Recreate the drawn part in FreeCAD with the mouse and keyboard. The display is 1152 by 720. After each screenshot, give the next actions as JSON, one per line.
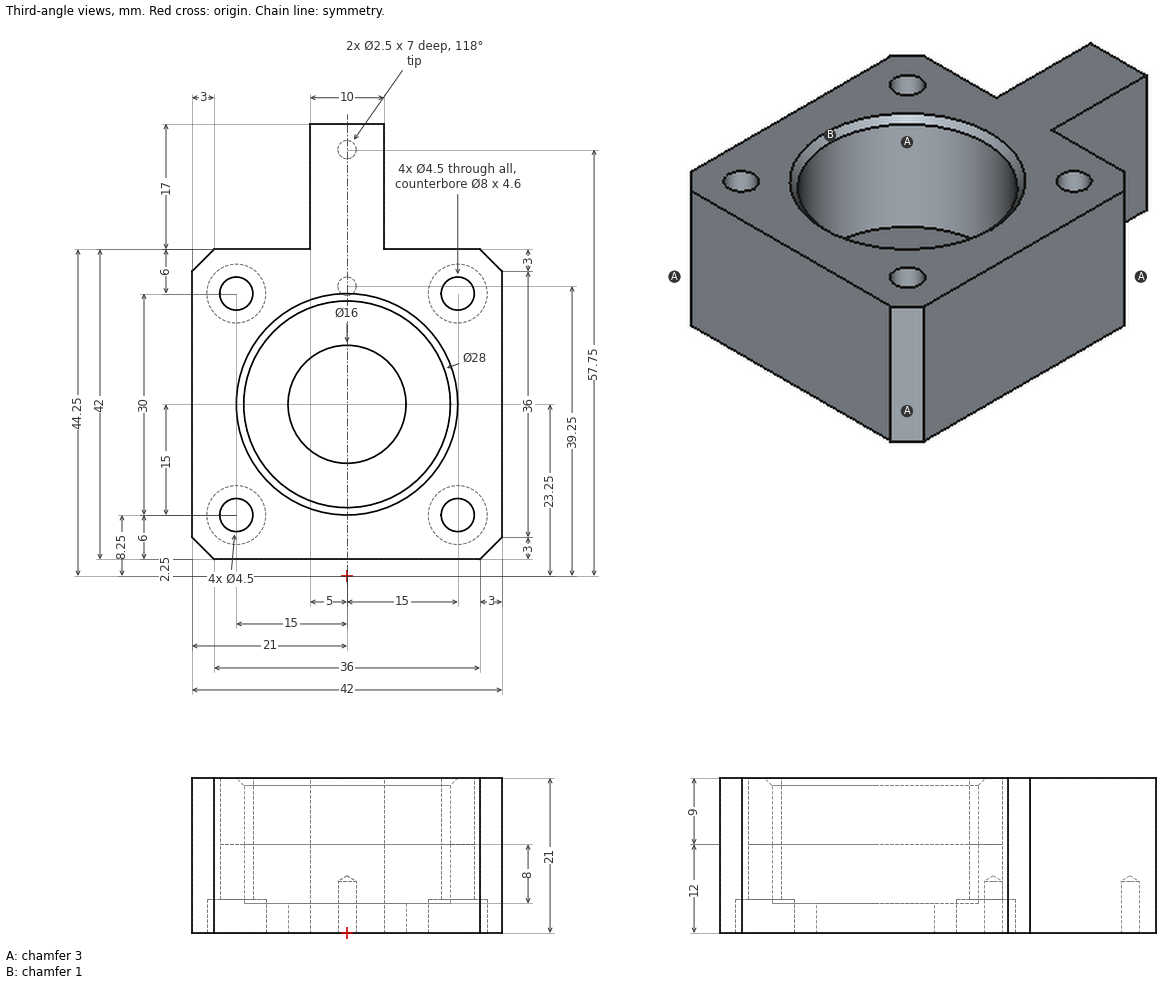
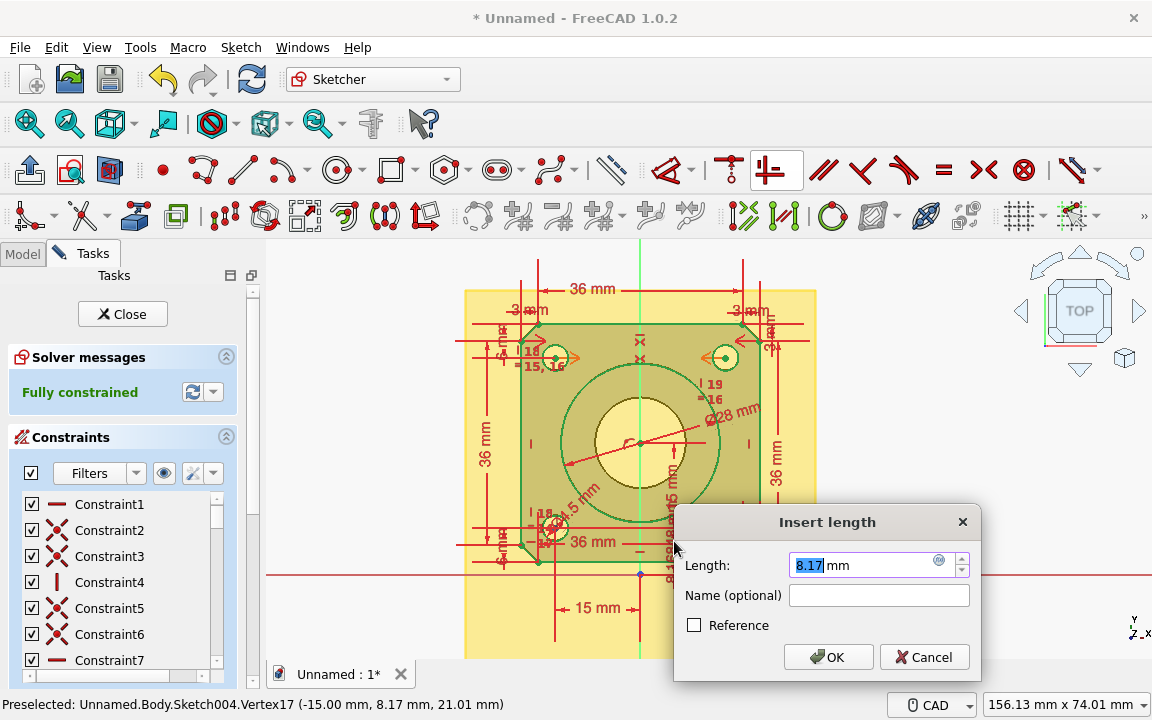
{"action": "type", "text": "8.25"}
{"action": "key", "text": "Return"}
{"action": "key", "text": "Escape"}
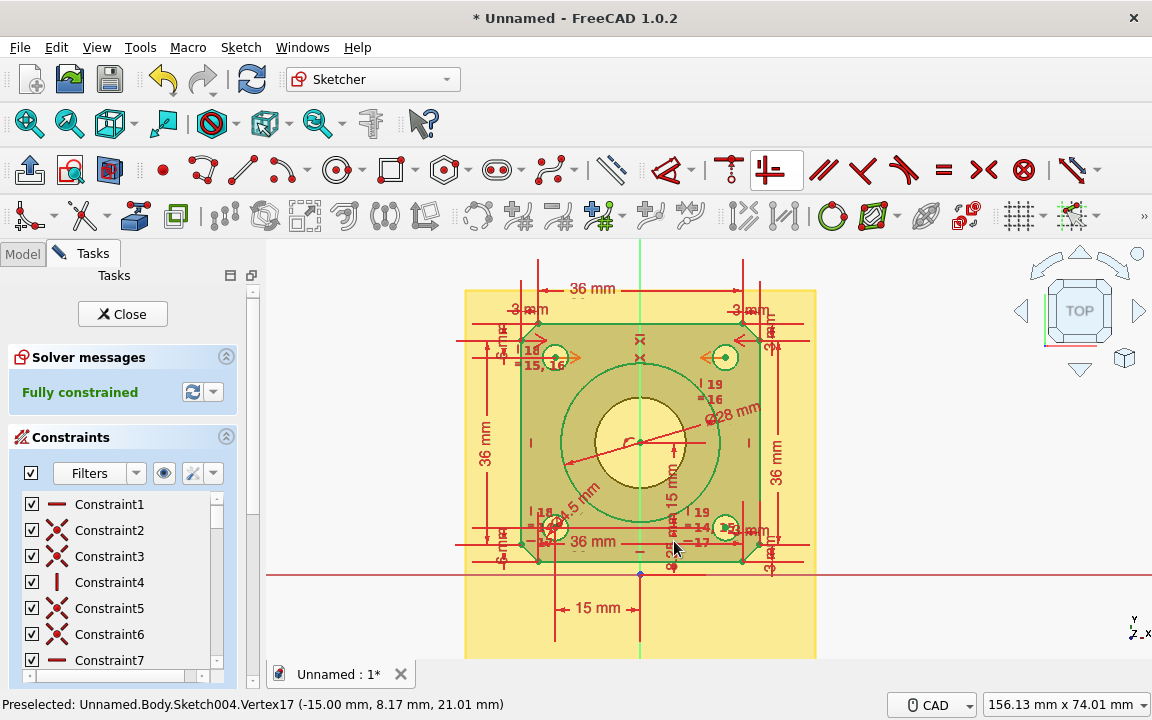
{"action": "left_click", "coordinate": [123, 314]}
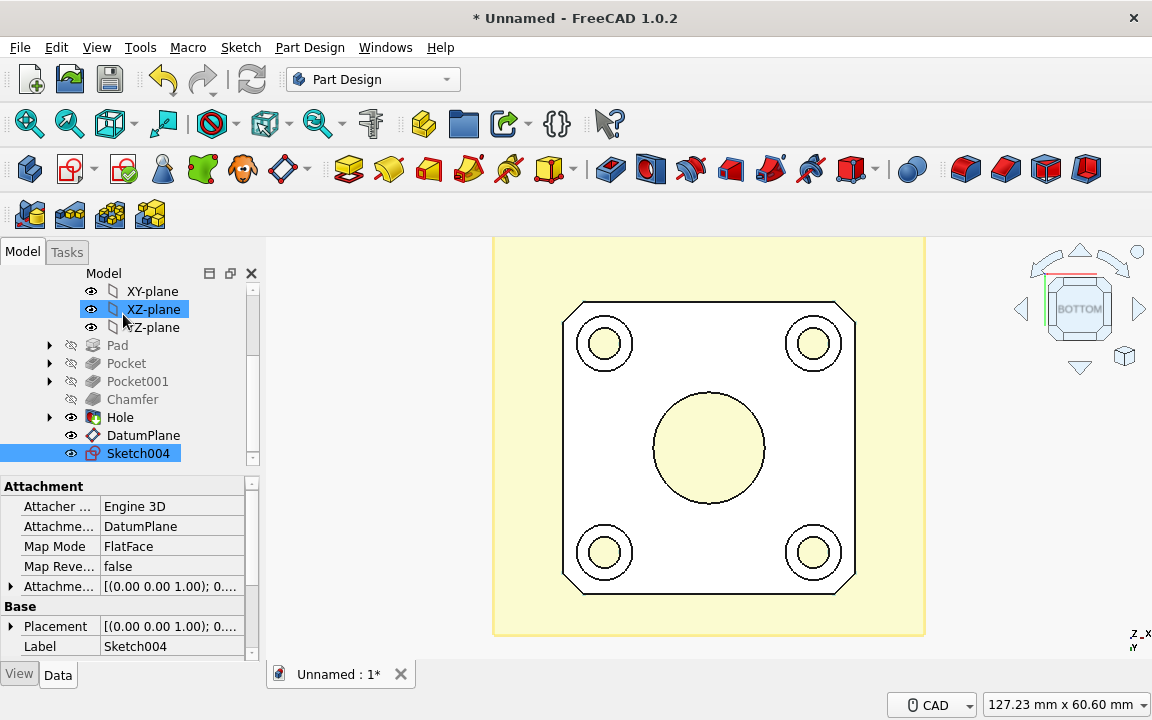
{"action": "left_click", "coordinate": [350, 170]}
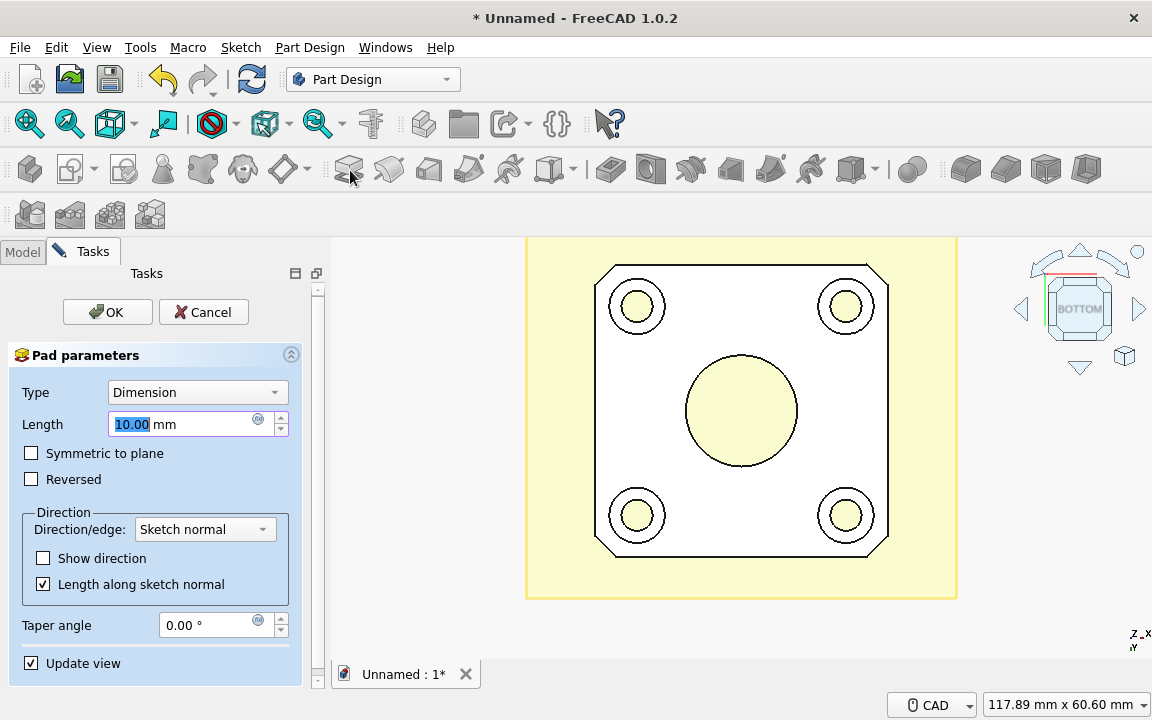
{"action": "type", "text": "9"}
{"action": "key", "text": "Tab"}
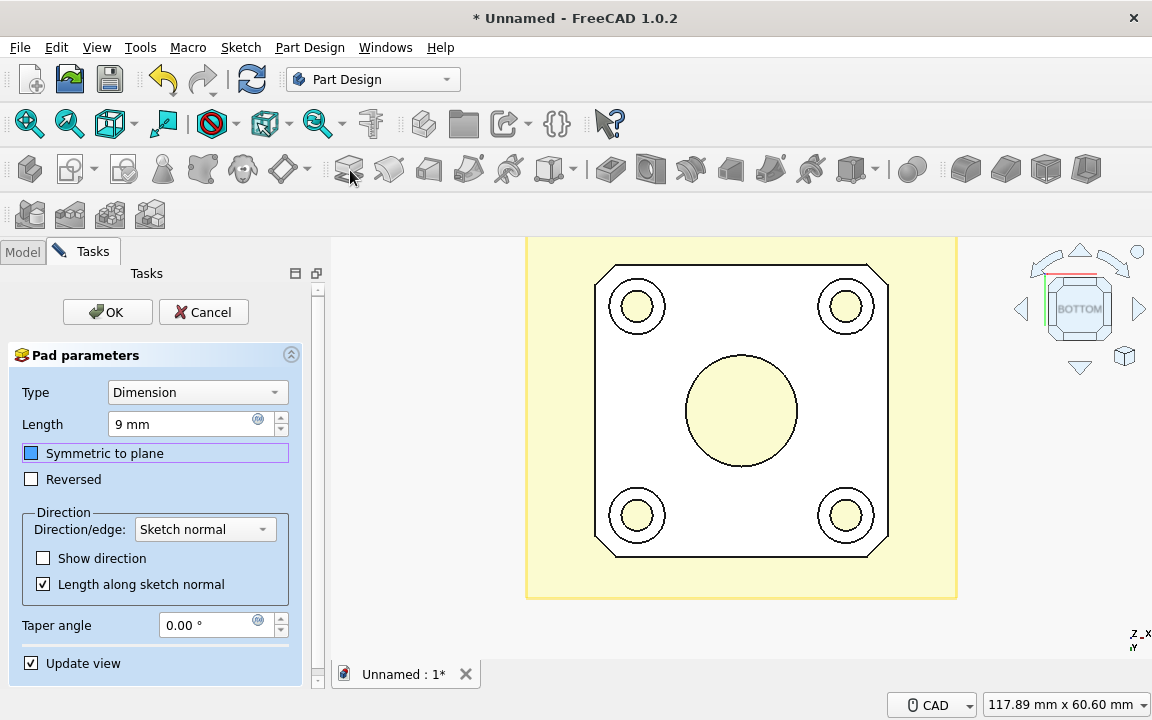
{"action": "left_click", "coordinate": [30, 479]}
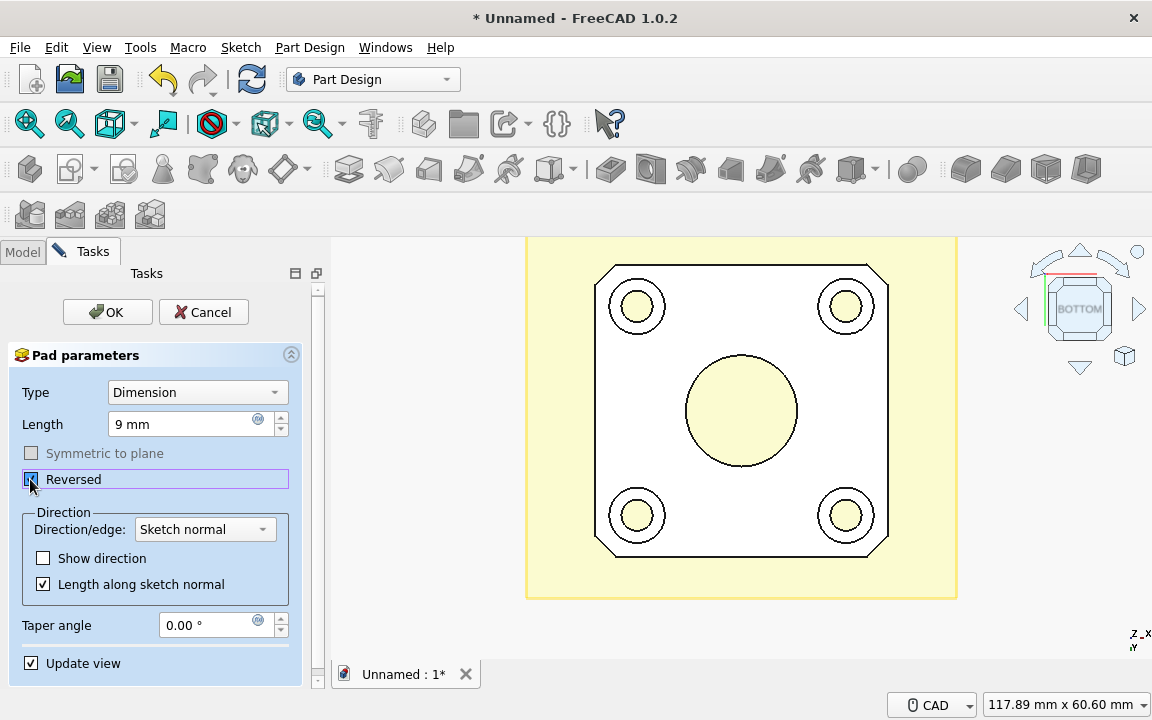
{"action": "left_click", "coordinate": [108, 312]}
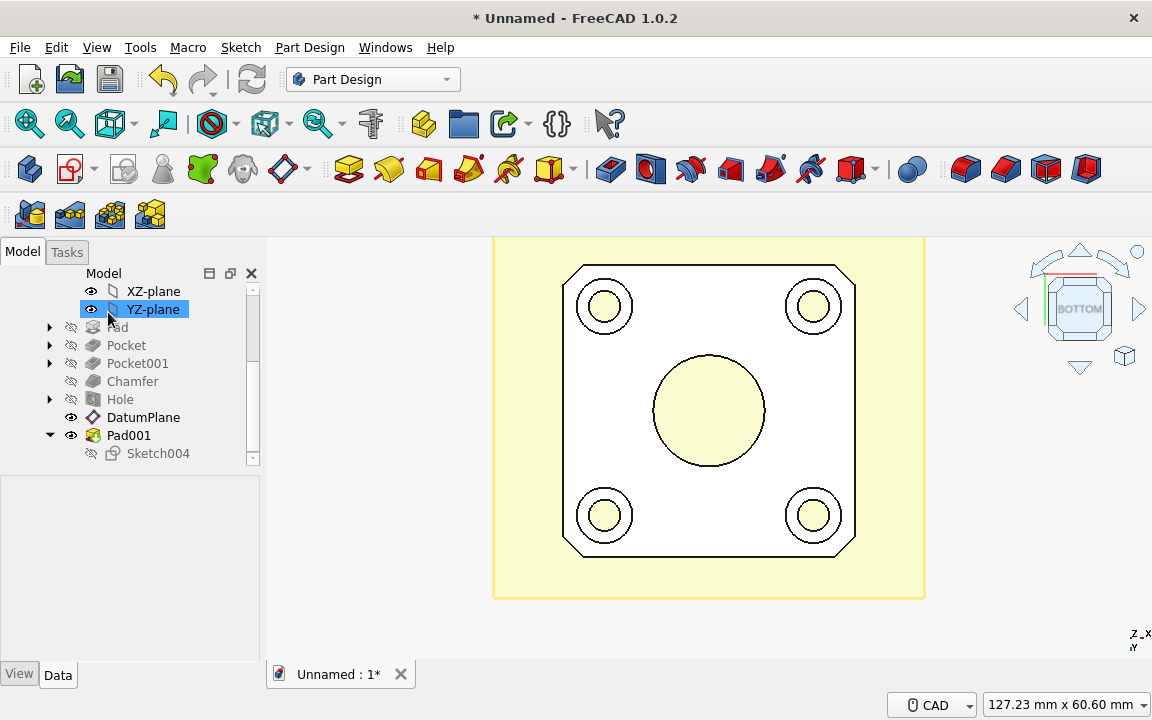
{"action": "left_click", "coordinate": [116, 417]}
{"action": "key", "text": "space"}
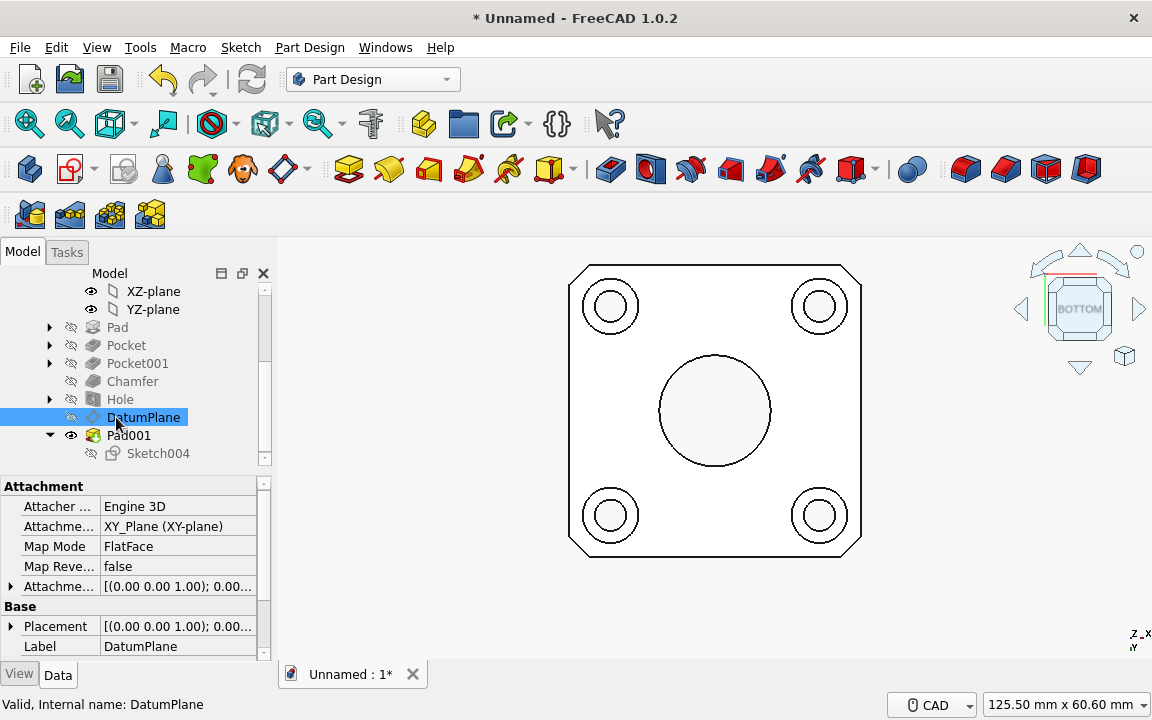
{"action": "left_click", "coordinate": [757, 326]}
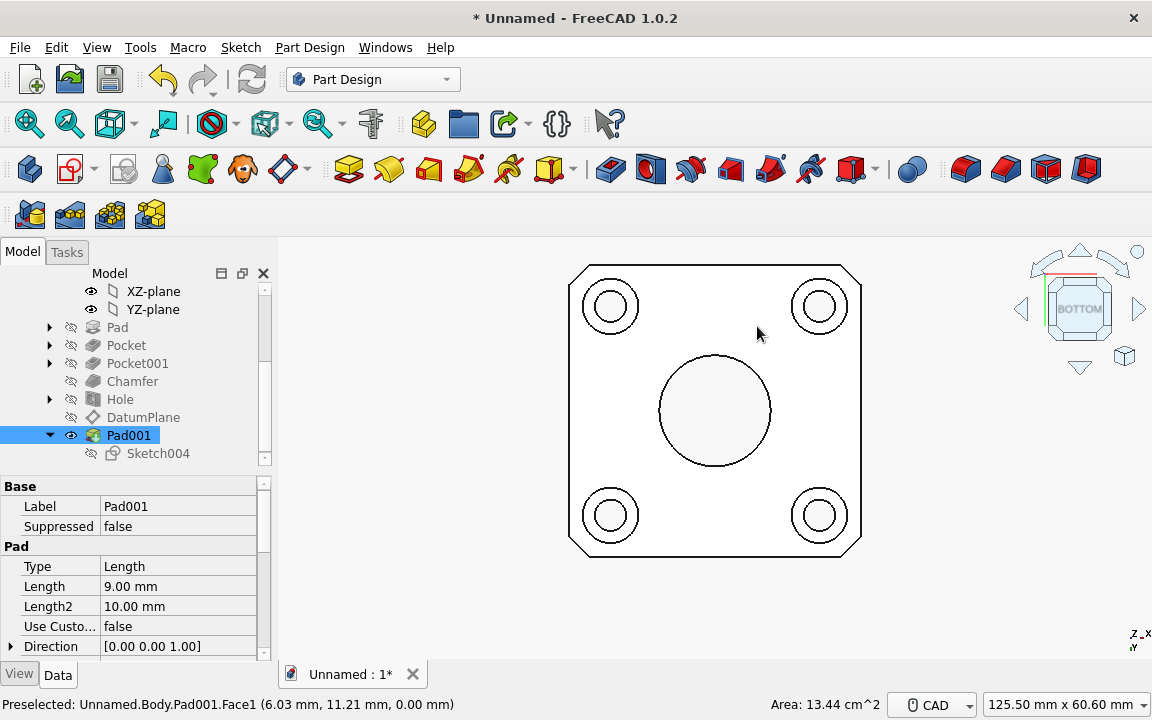
{"action": "left_click", "coordinate": [70, 170]}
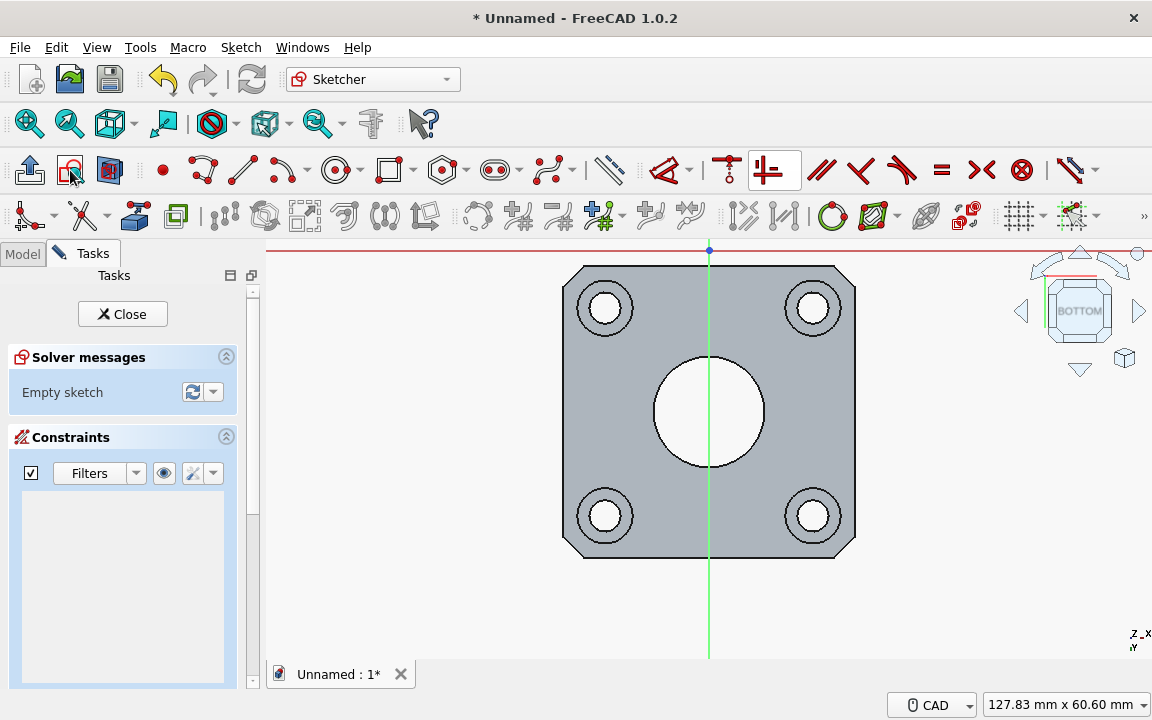
{"action": "scroll", "coordinate": [640, 449], "scroll_direction": "down", "scroll_amount": 5}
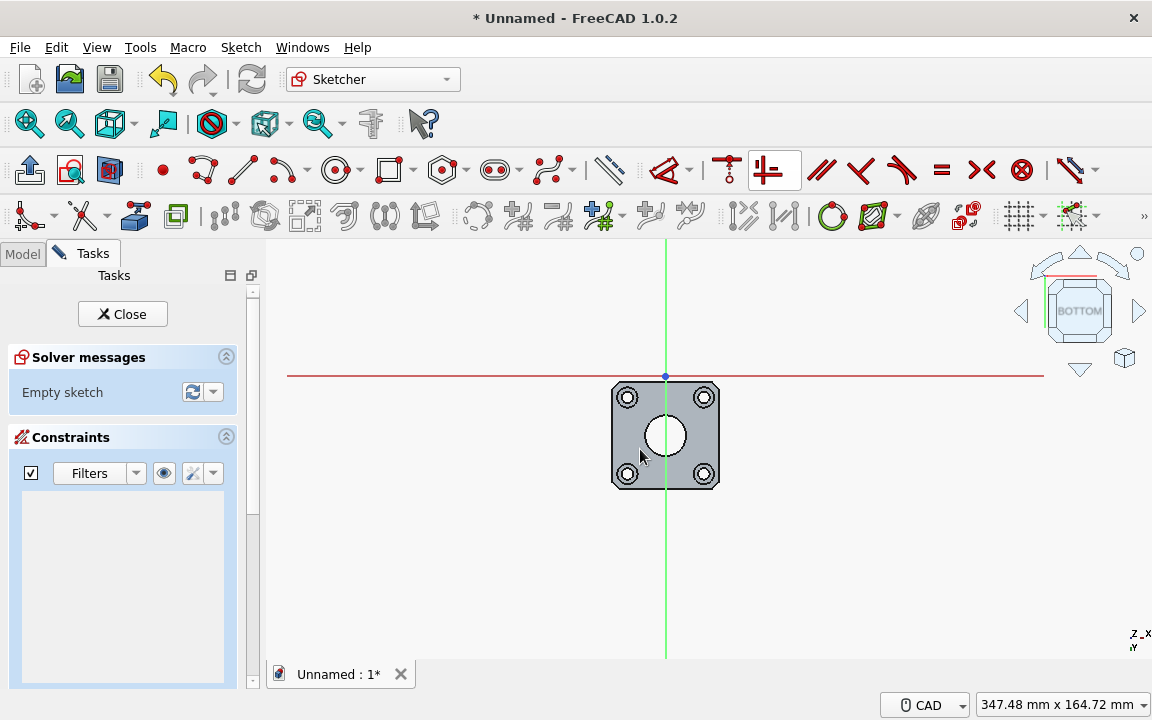
{"action": "scroll", "coordinate": [671, 523], "scroll_direction": "up", "scroll_amount": 9}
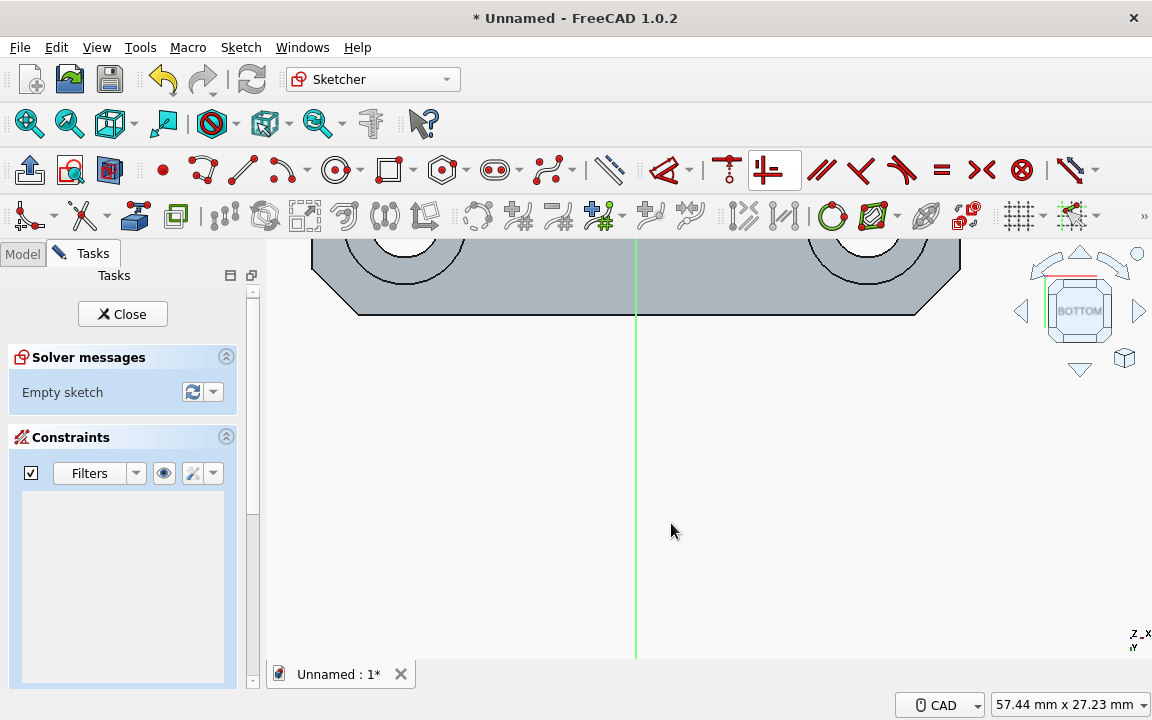
{"action": "left_click", "coordinate": [390, 170]}